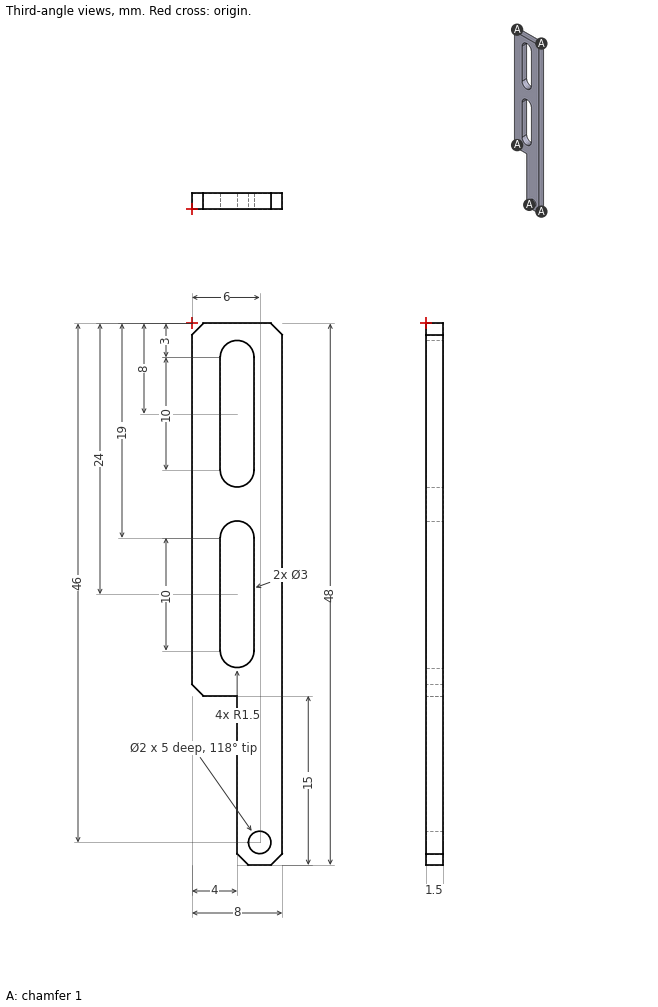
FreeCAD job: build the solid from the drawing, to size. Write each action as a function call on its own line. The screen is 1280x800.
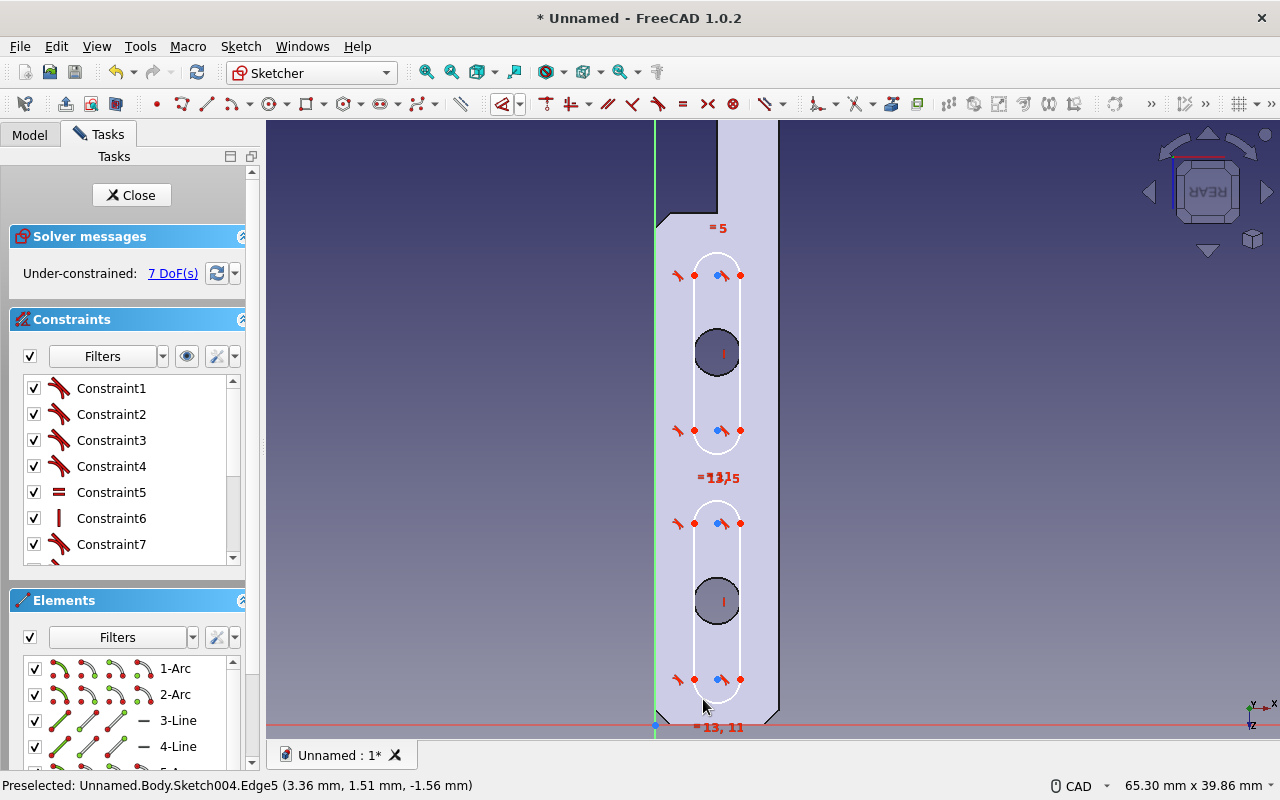
scroll(703, 450, up, 3)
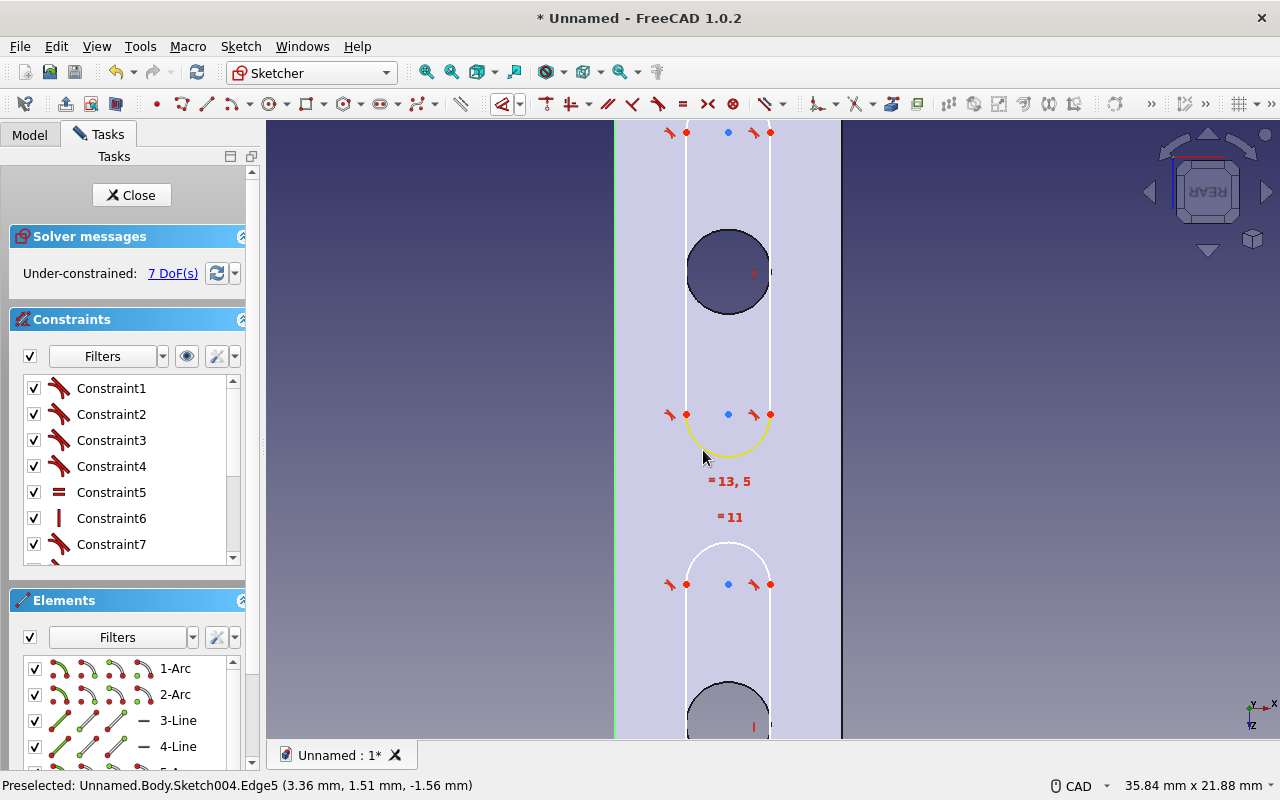
click(704, 449)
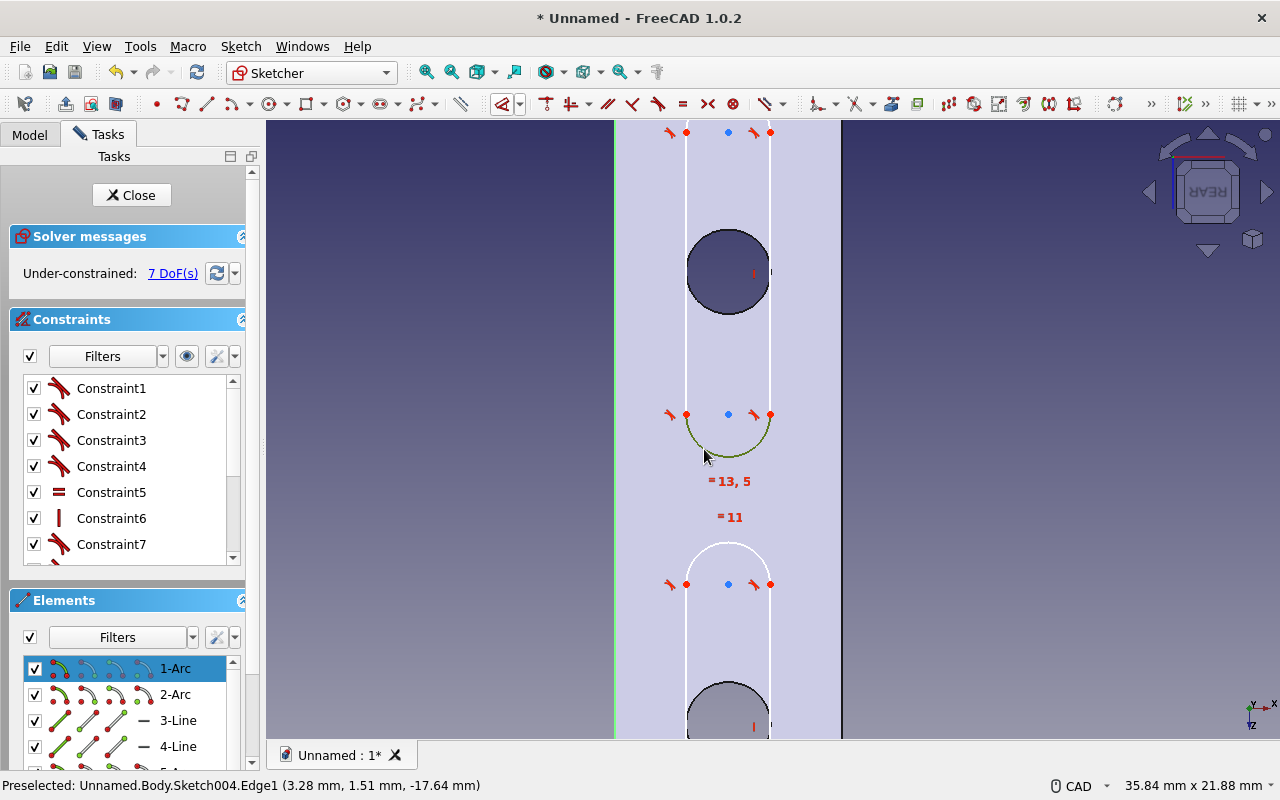
key(k)
key(r)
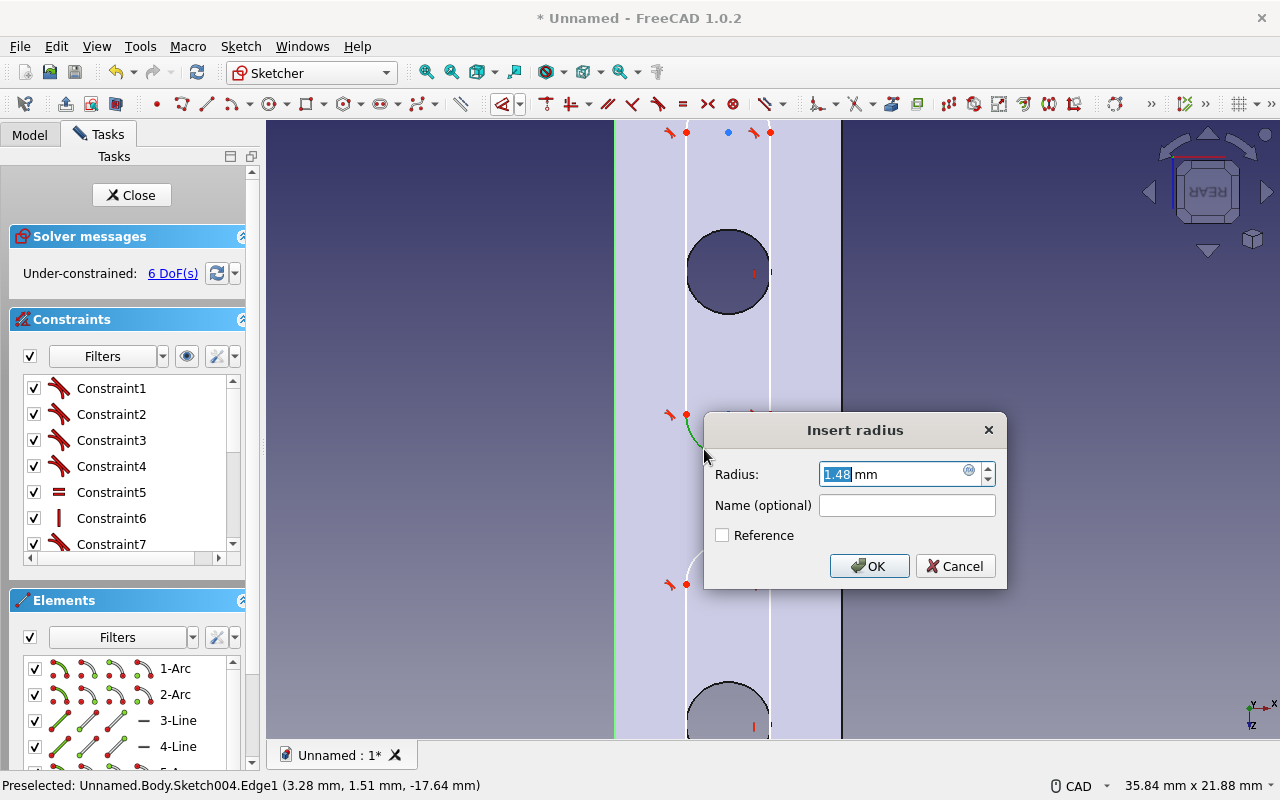
text(1.5)
key(Return)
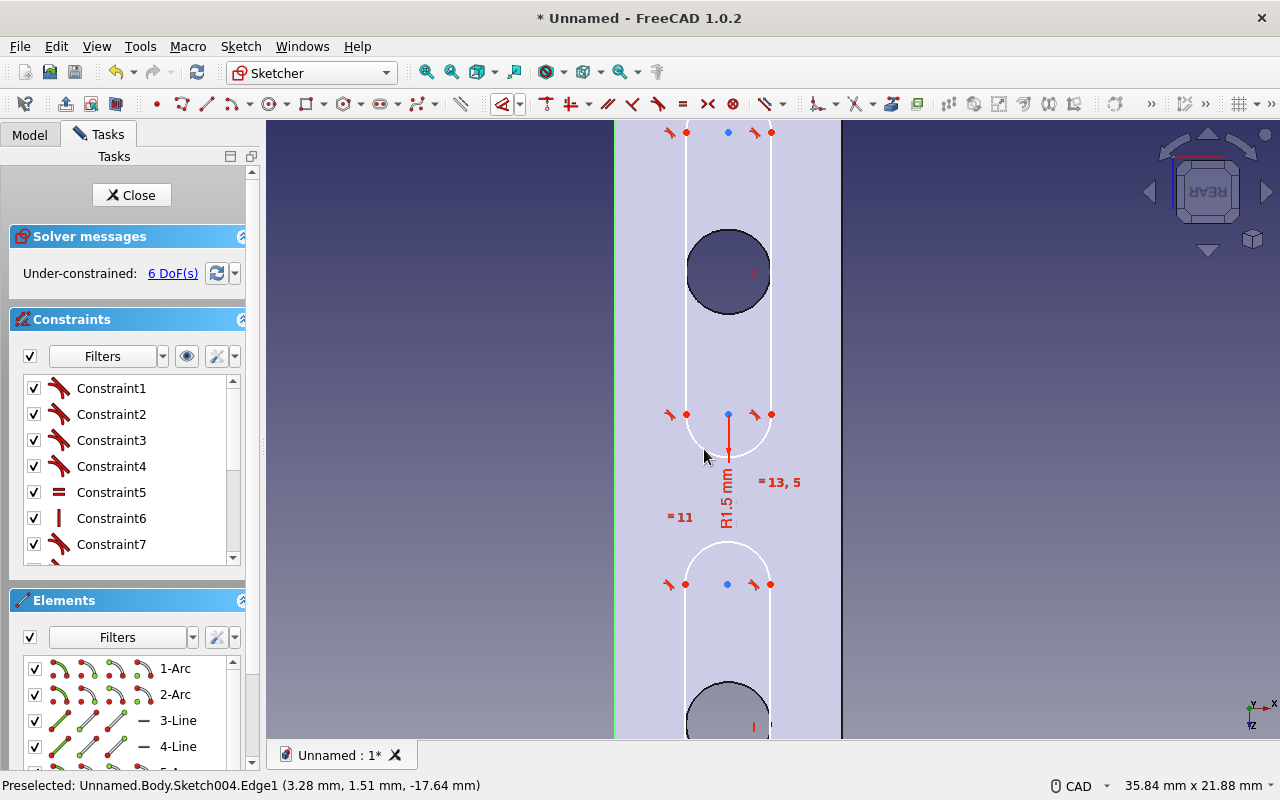
click(686, 330)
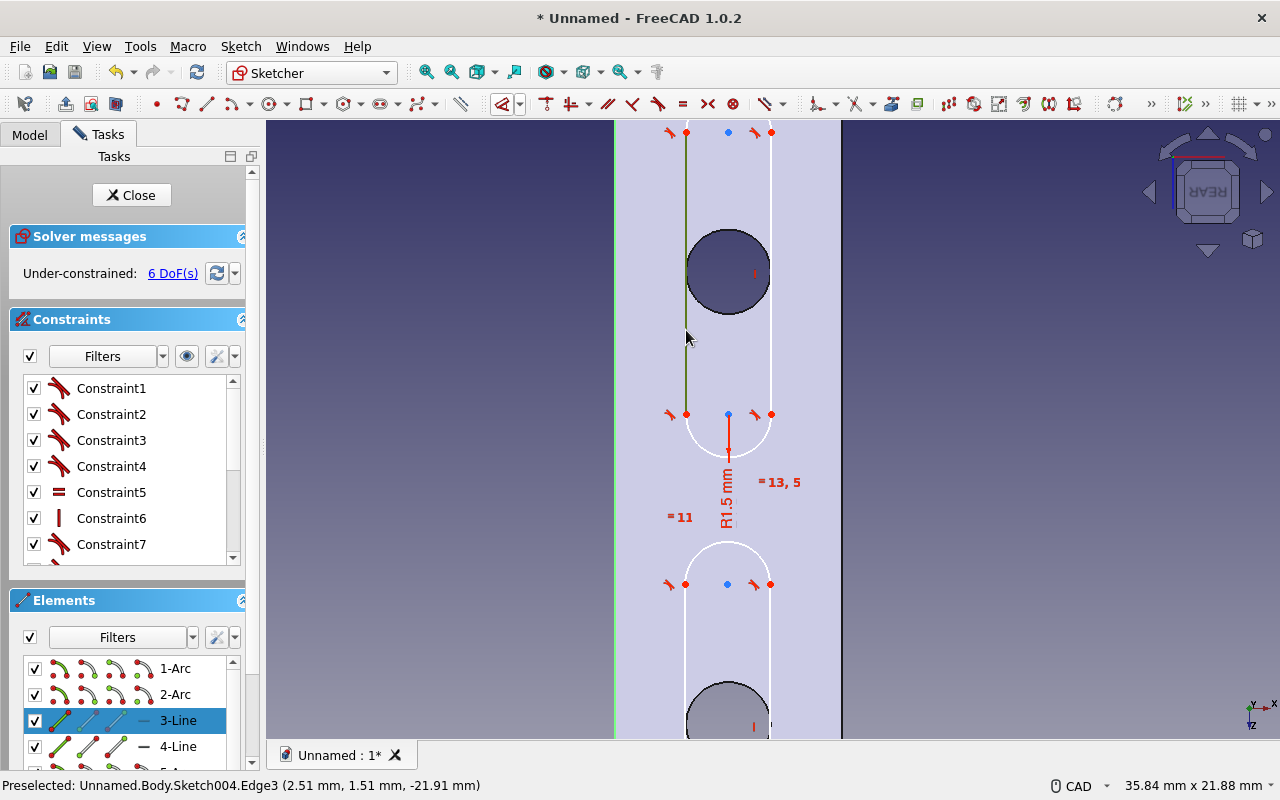
key(i)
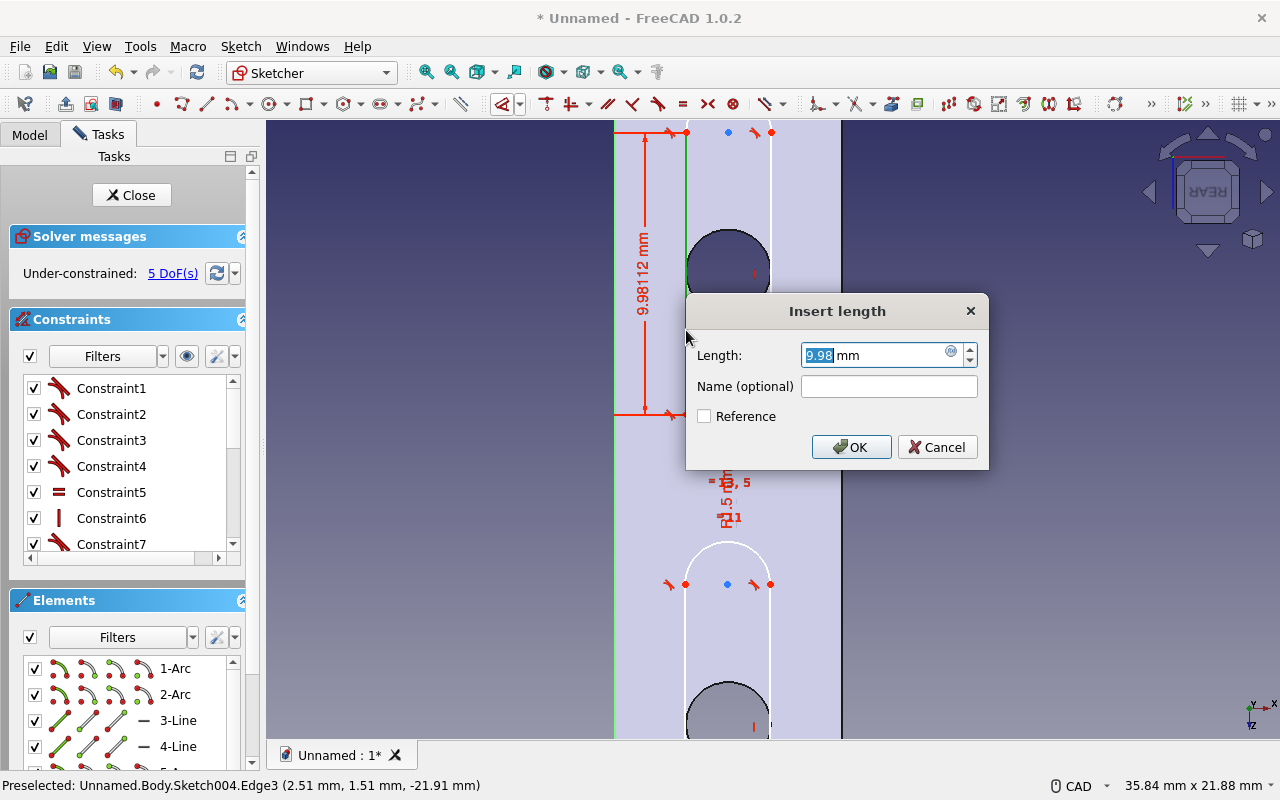
text(10)
key(Return)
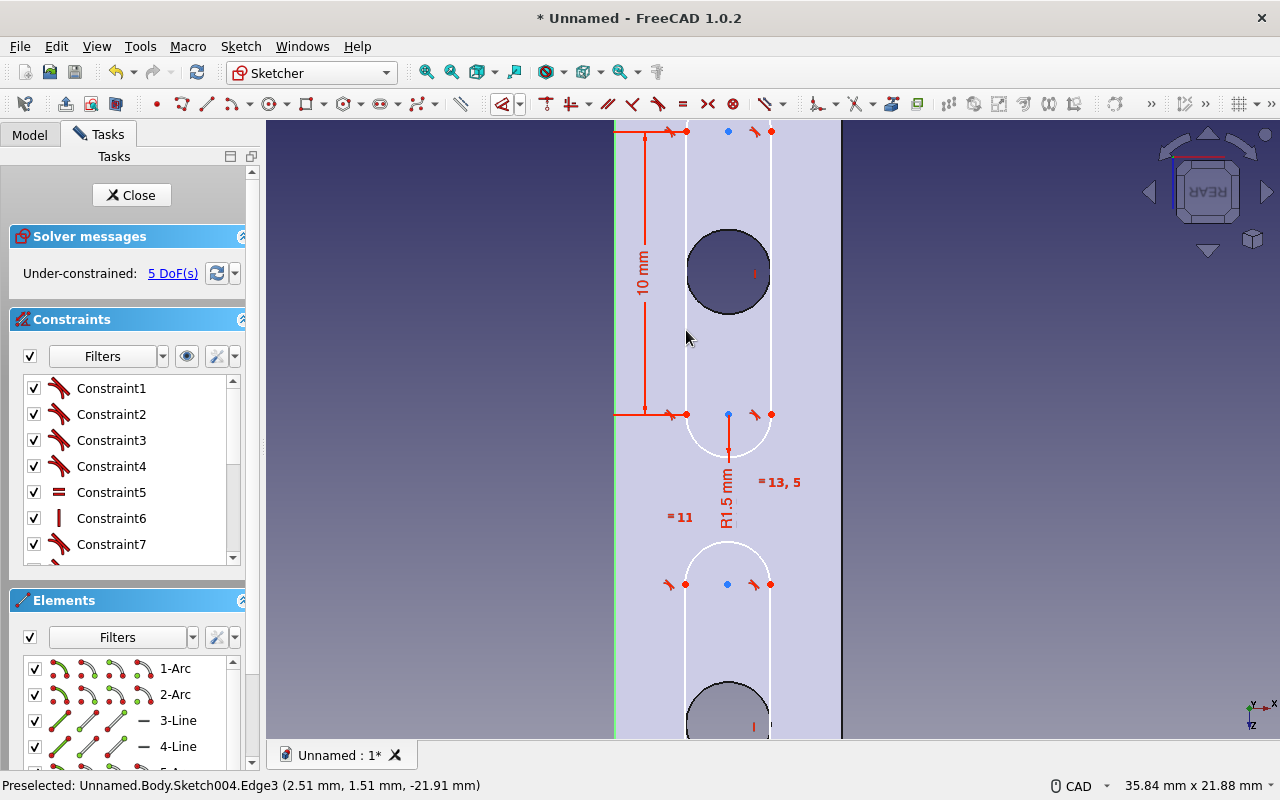
click(685, 670)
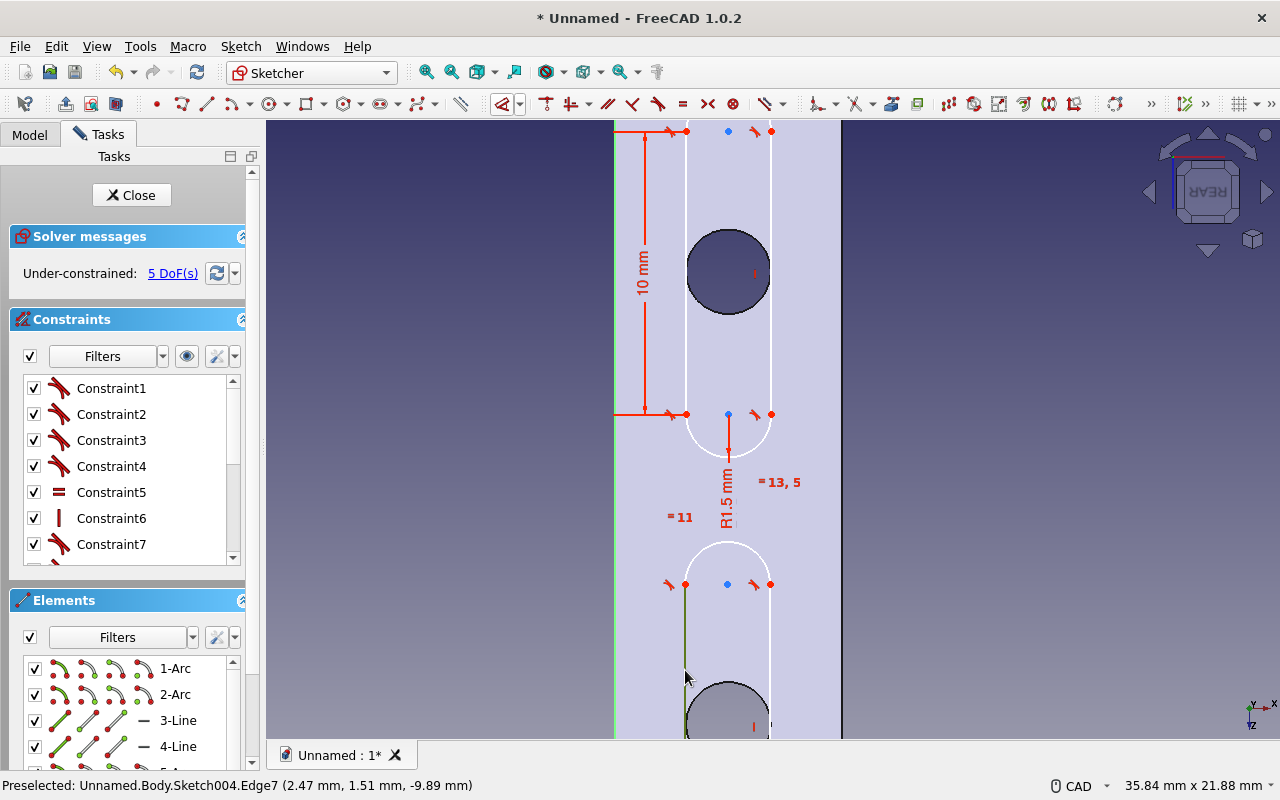
key(i)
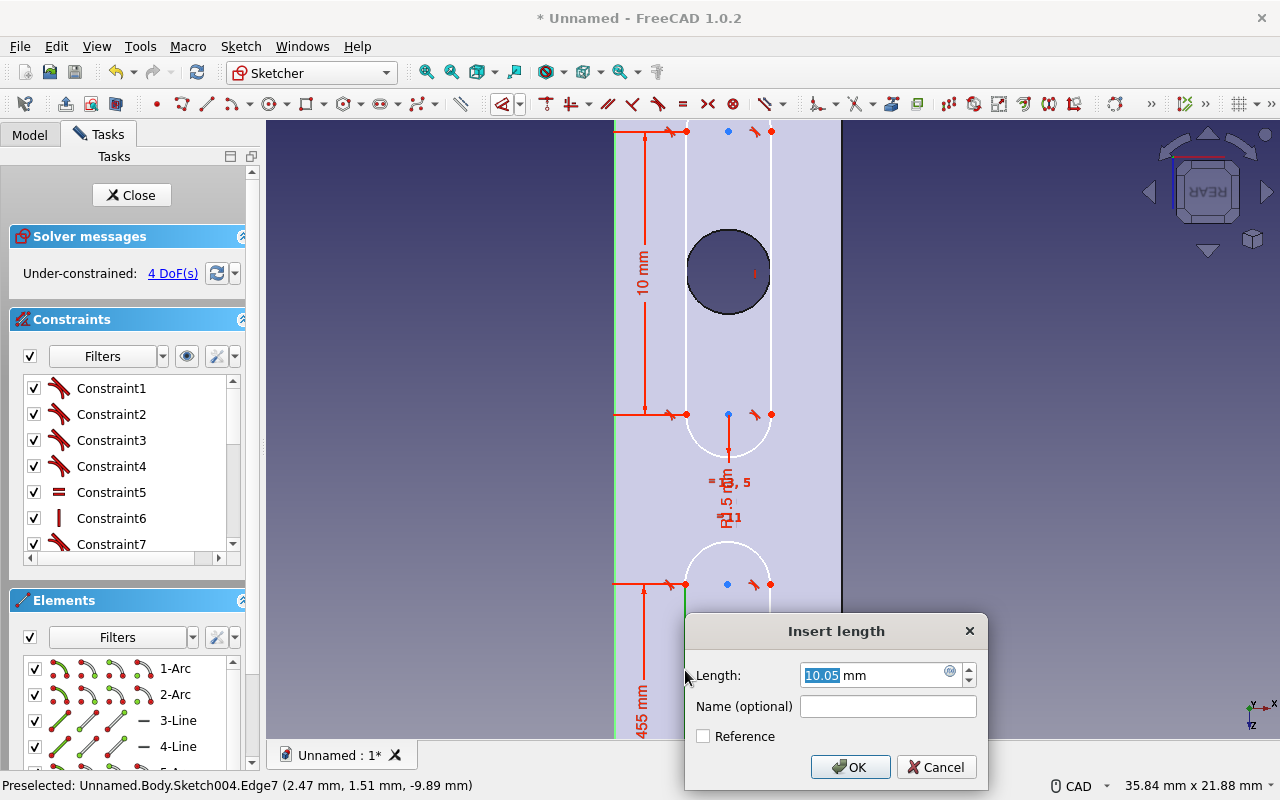
text(10)
key(Return)